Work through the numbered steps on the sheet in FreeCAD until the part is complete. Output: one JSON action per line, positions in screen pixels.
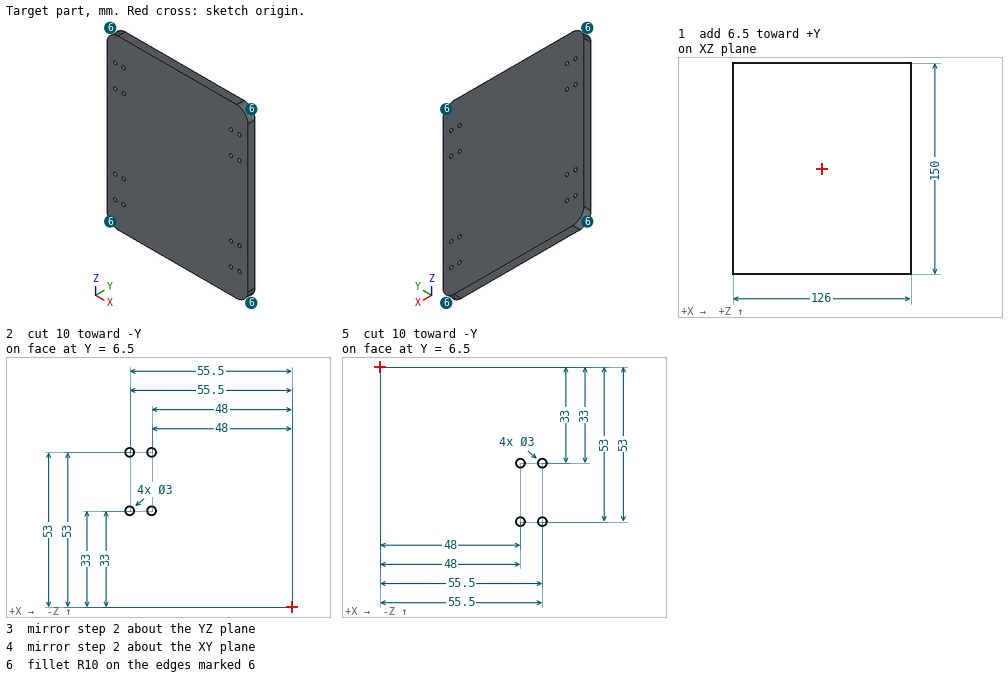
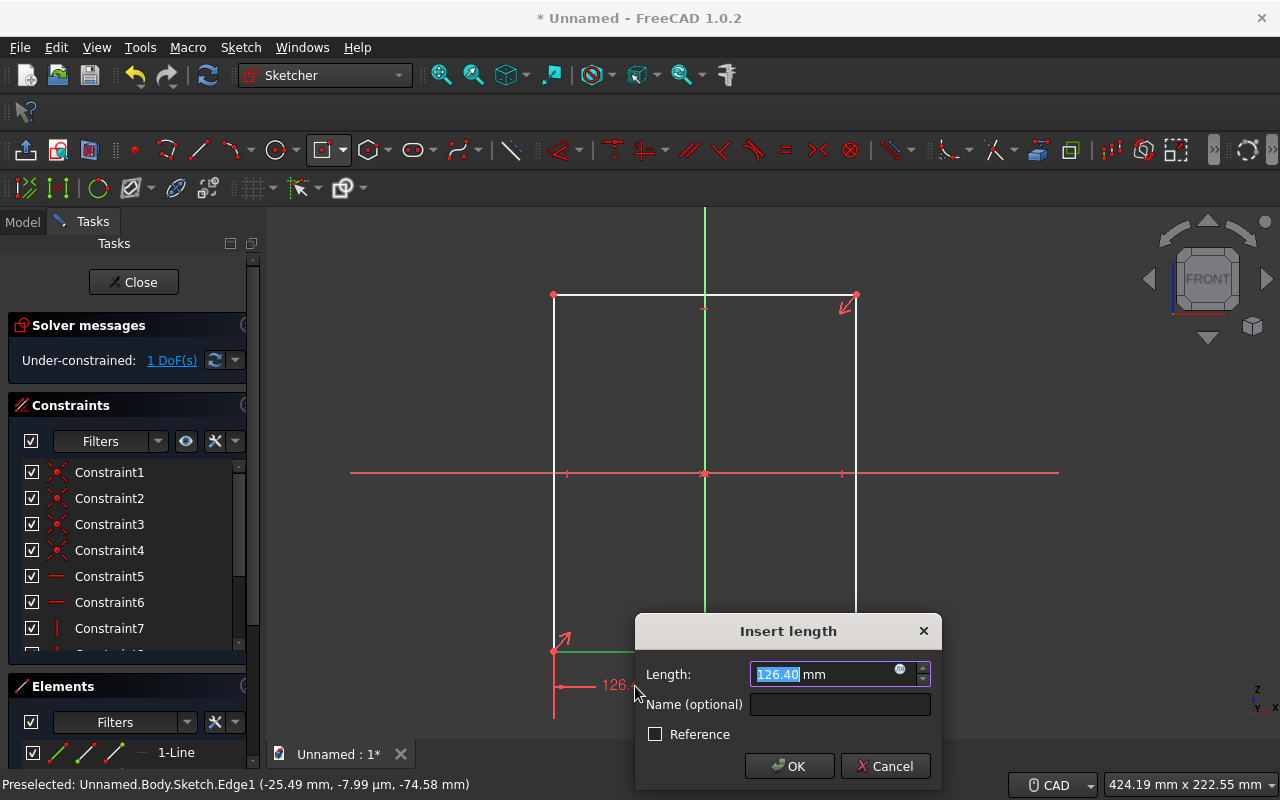
{"action": "type", "text": "126"}
{"action": "key", "text": "Return"}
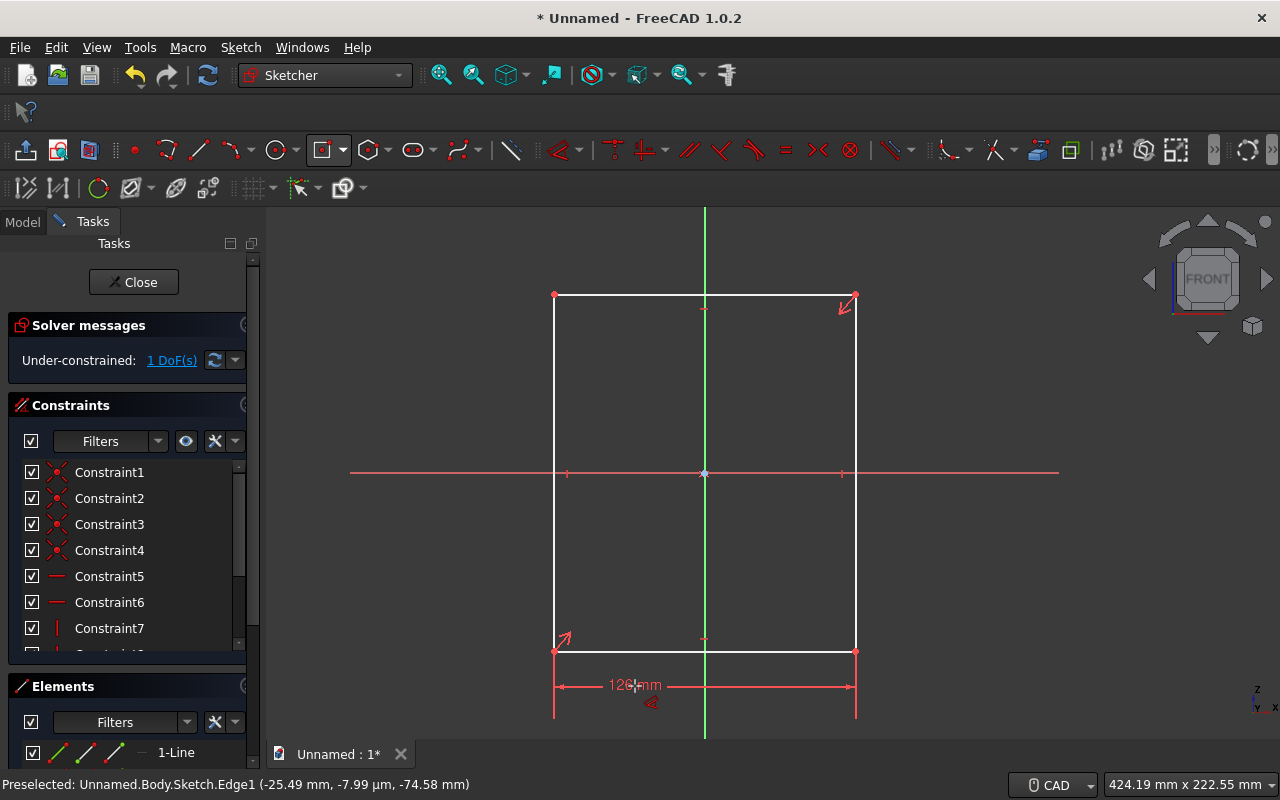
{"action": "left_click", "coordinate": [856, 545]}
{"action": "left_click", "coordinate": [890, 391]}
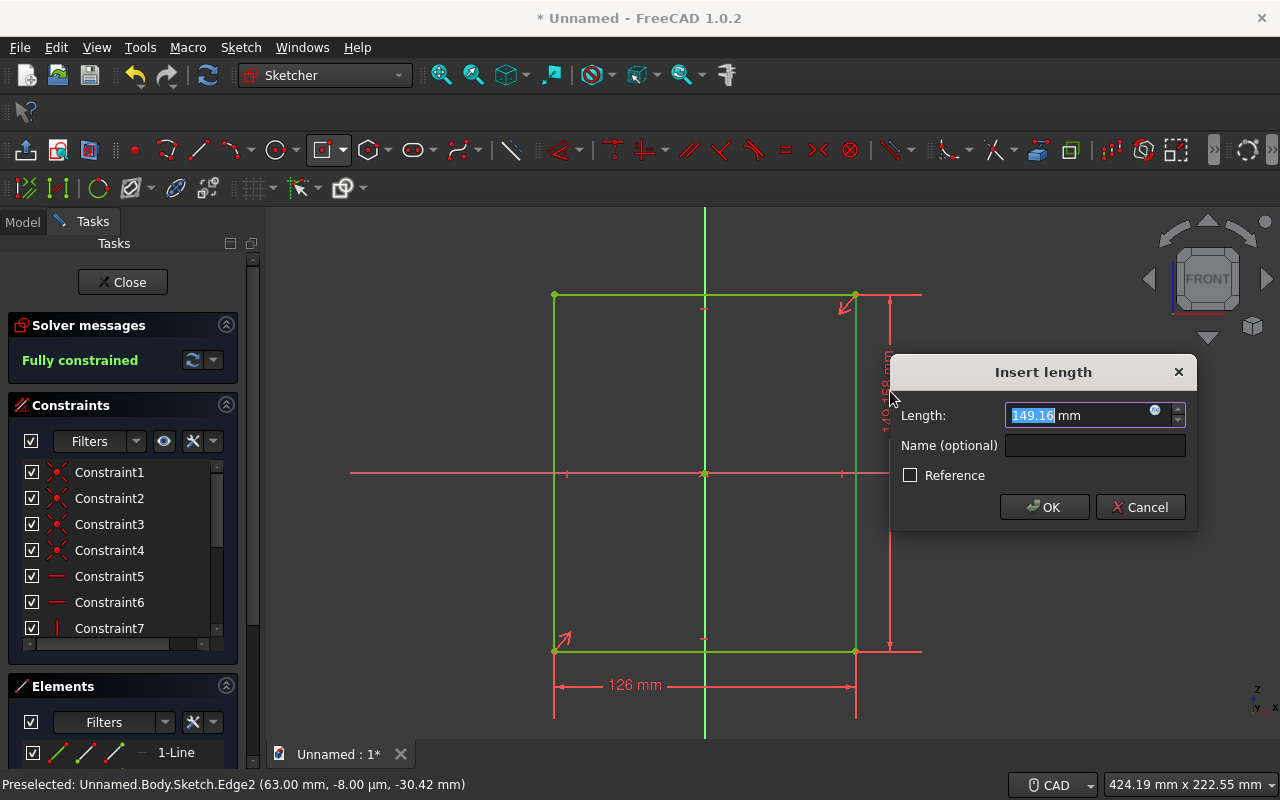
{"action": "type", "text": "150"}
{"action": "key", "text": "Return"}
{"action": "key", "text": "Escape"}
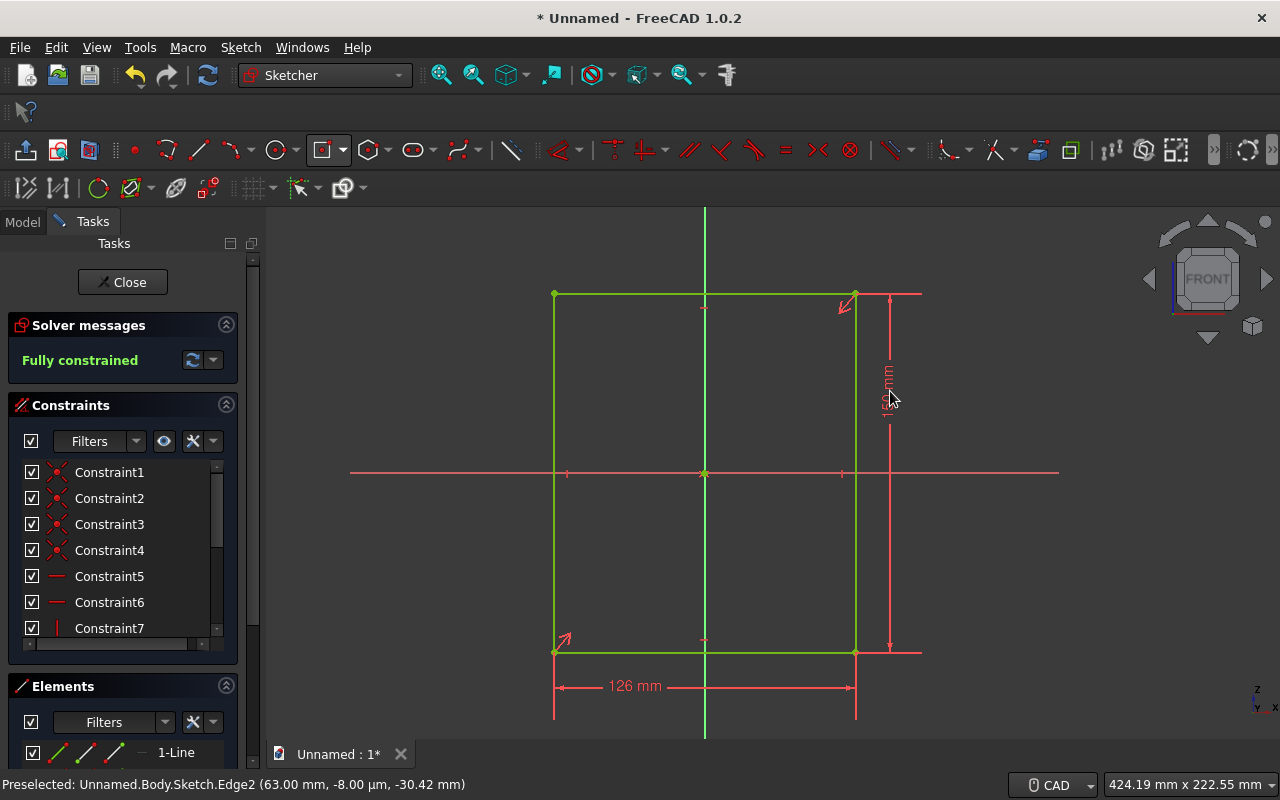
{"action": "left_click", "coordinate": [123, 282]}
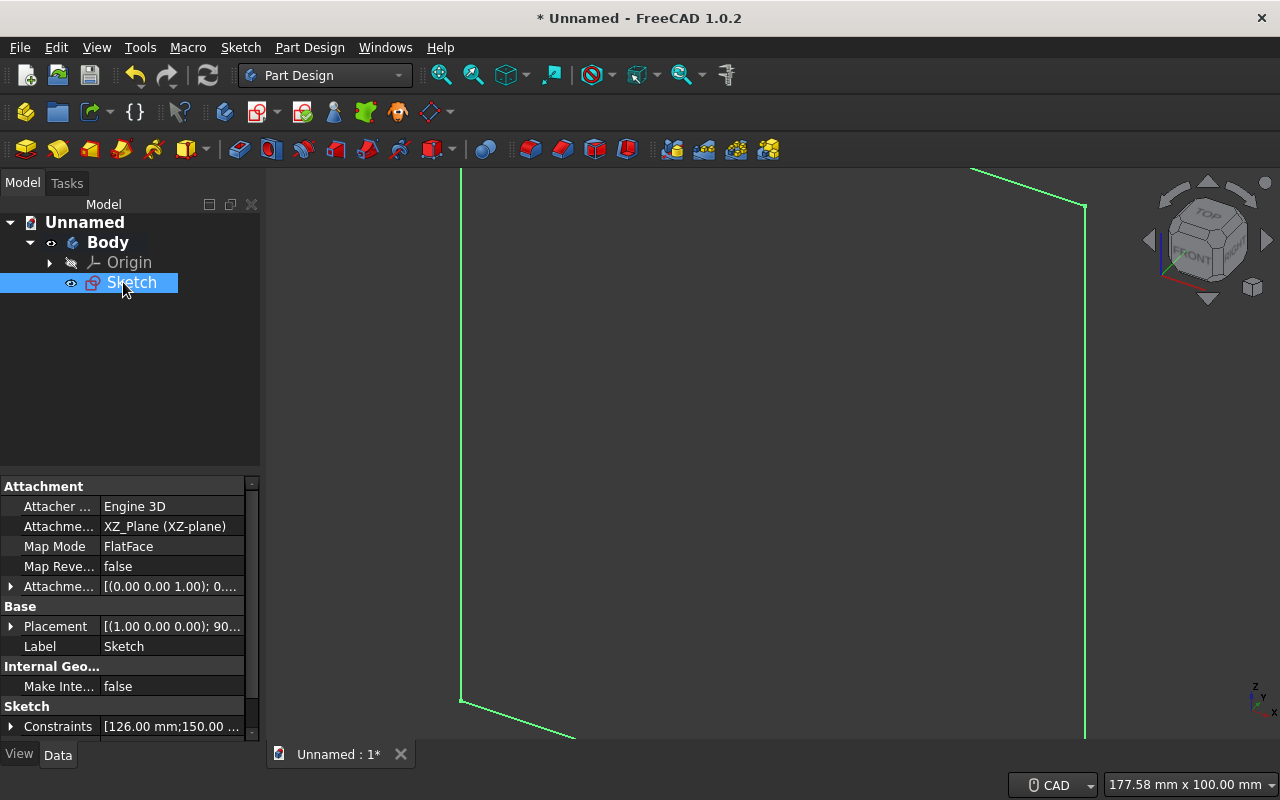
{"action": "left_click", "coordinate": [26, 150]}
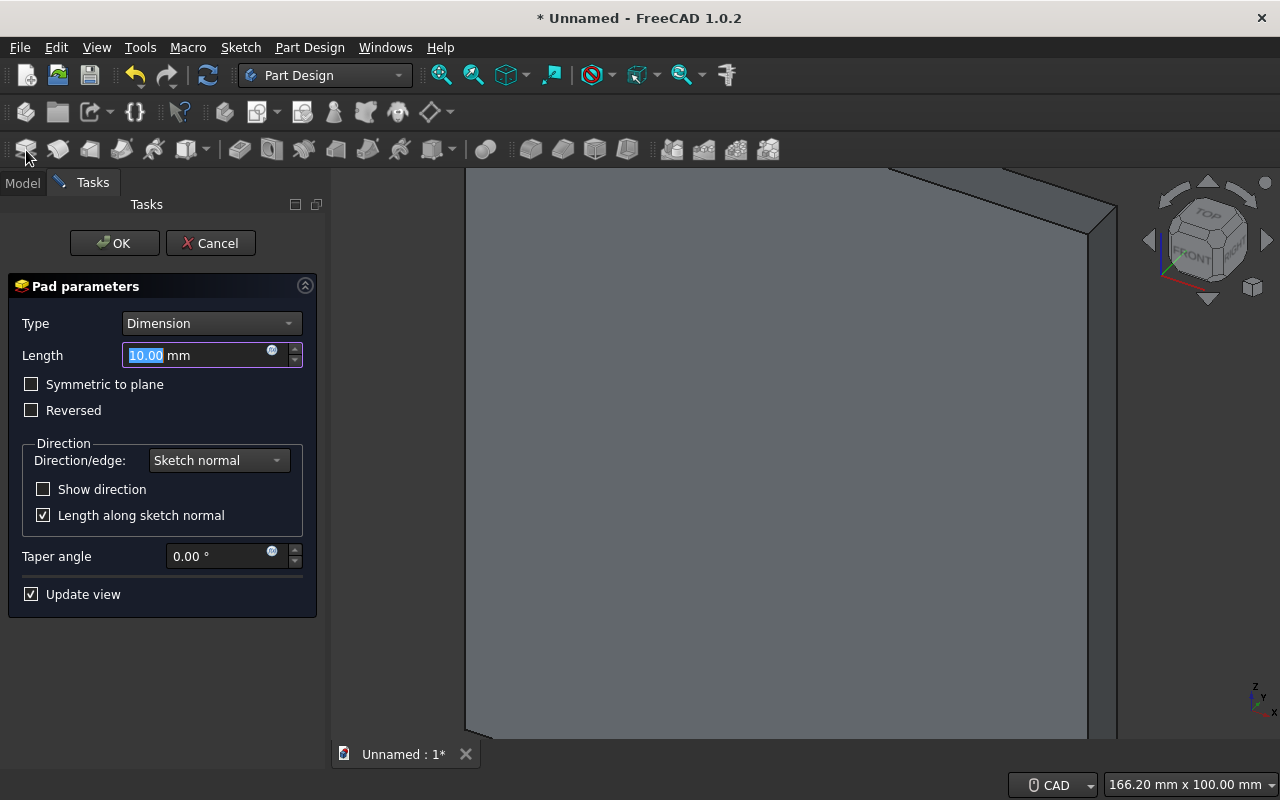
{"action": "type", "text": "6.5"}
{"action": "key", "text": "Tab"}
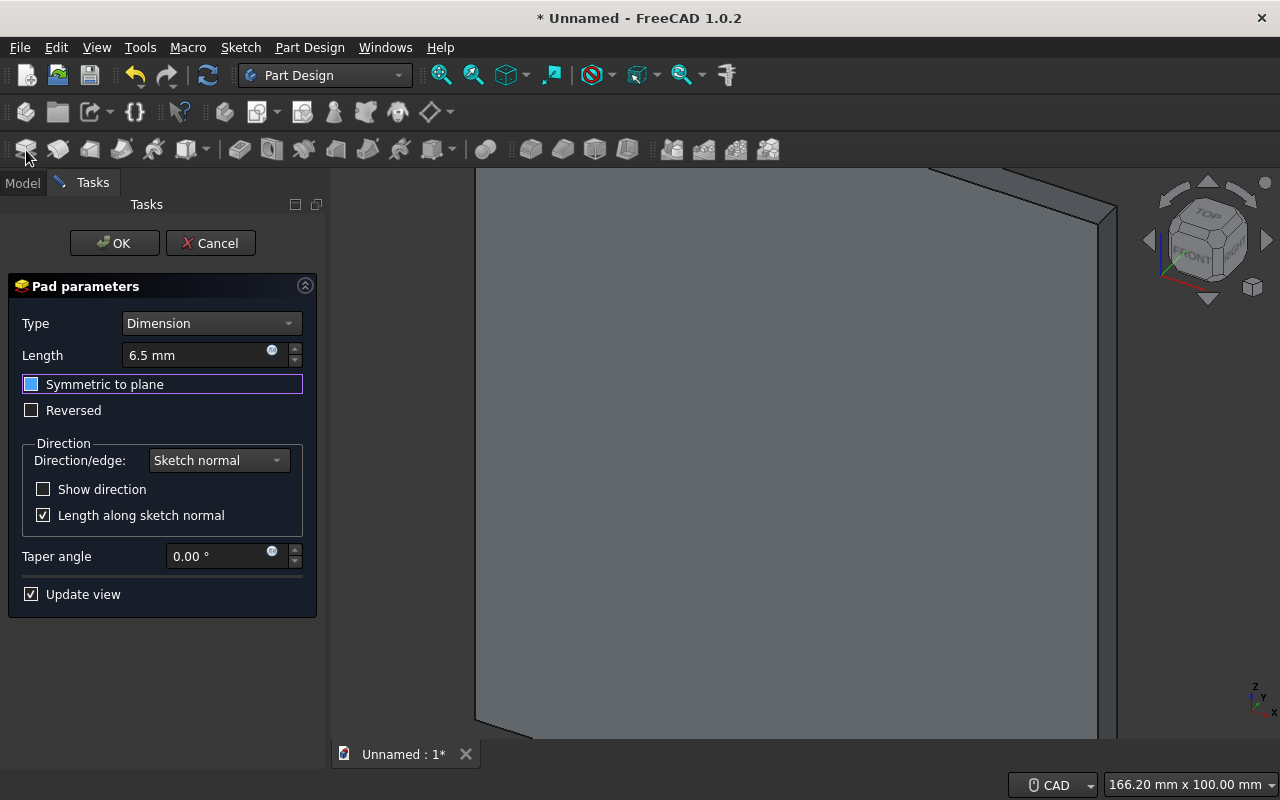
{"action": "left_click", "coordinate": [30, 410]}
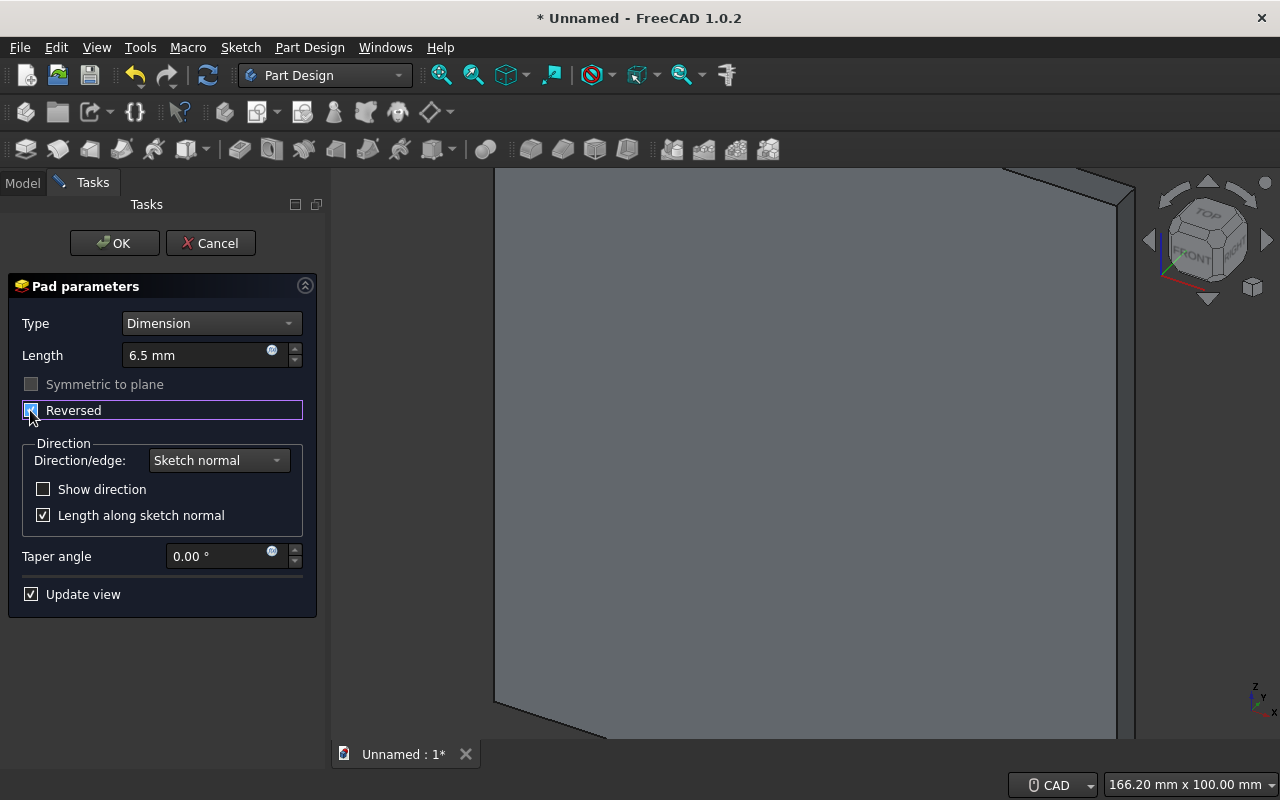
{"action": "left_click", "coordinate": [115, 243]}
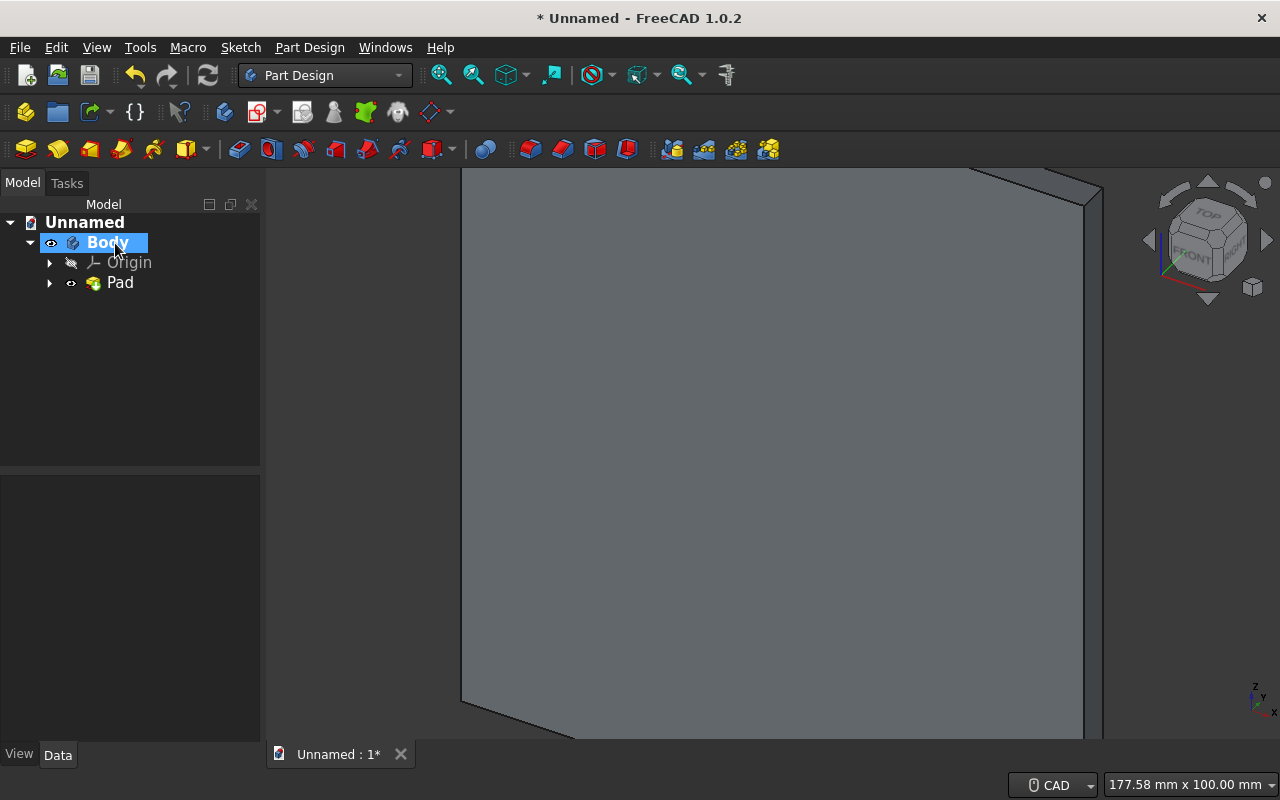
{"action": "left_click", "coordinate": [442, 76]}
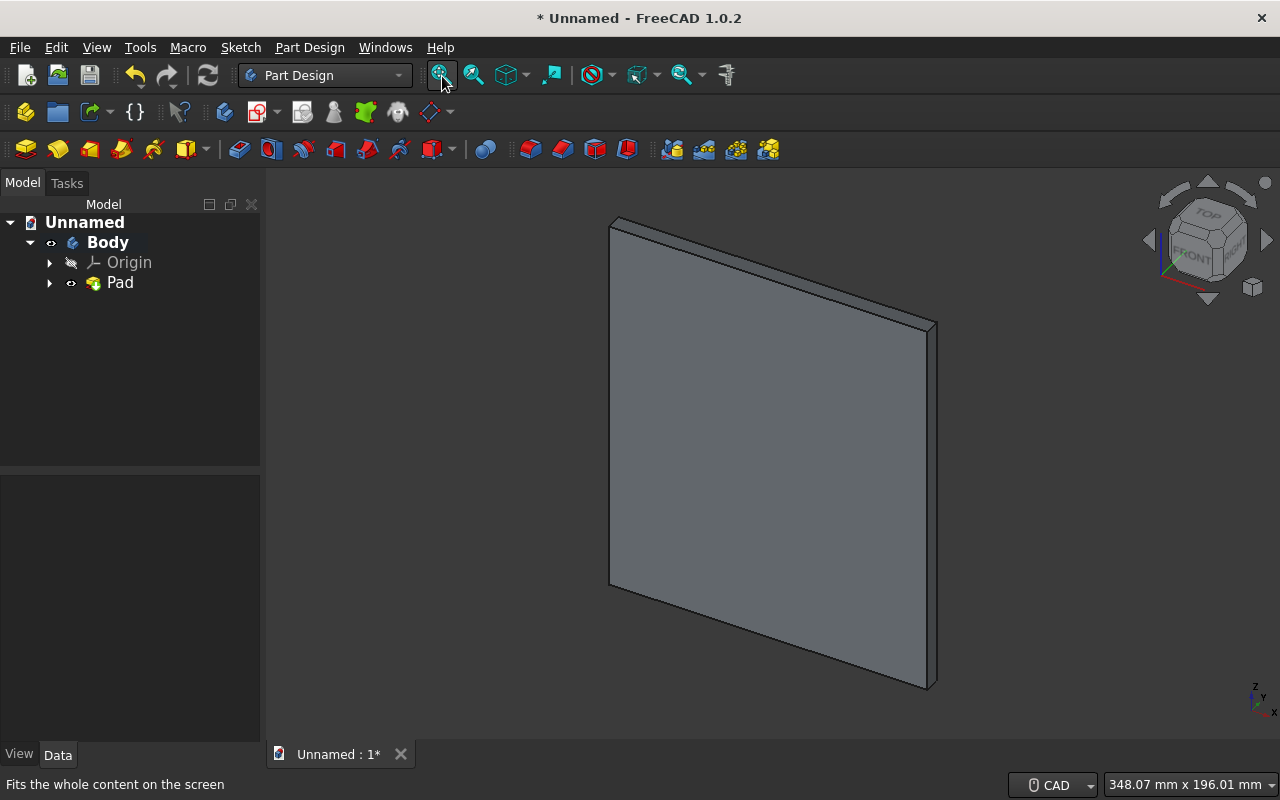
{"action": "key", "text": "4"}